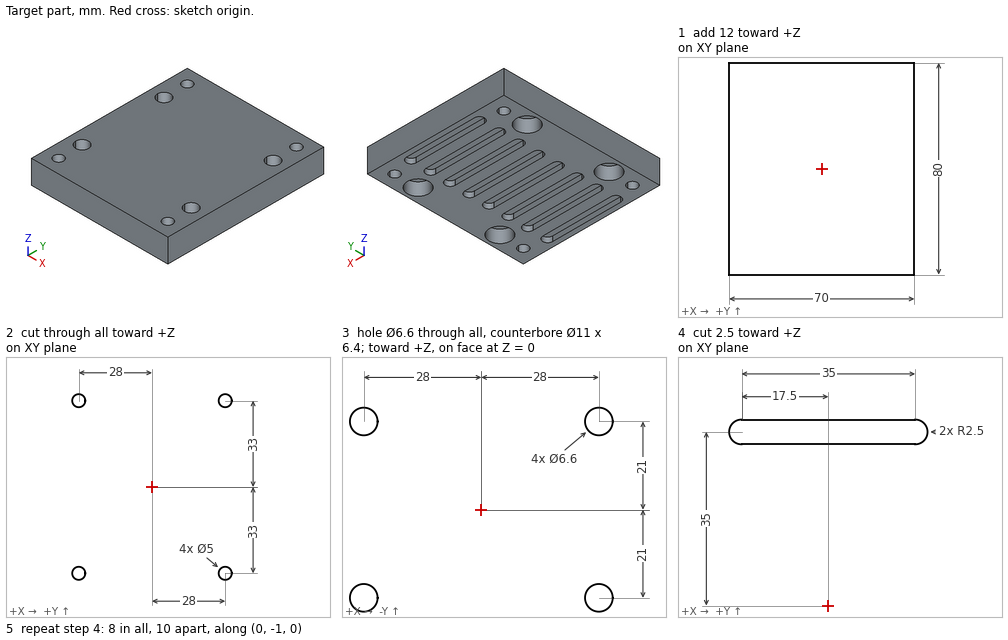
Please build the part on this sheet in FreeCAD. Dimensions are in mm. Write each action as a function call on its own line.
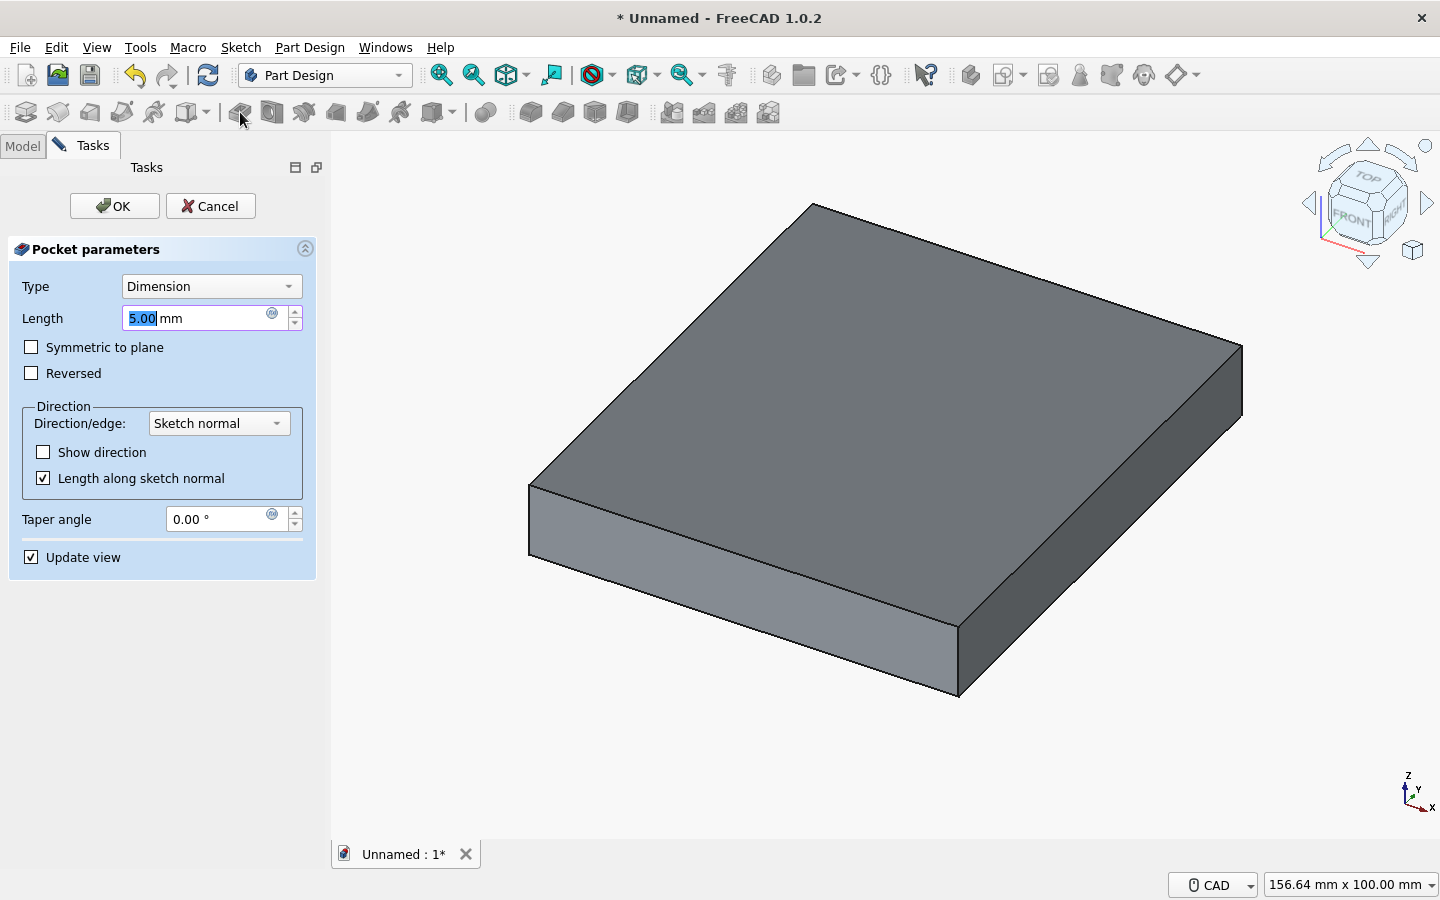
click(212, 286)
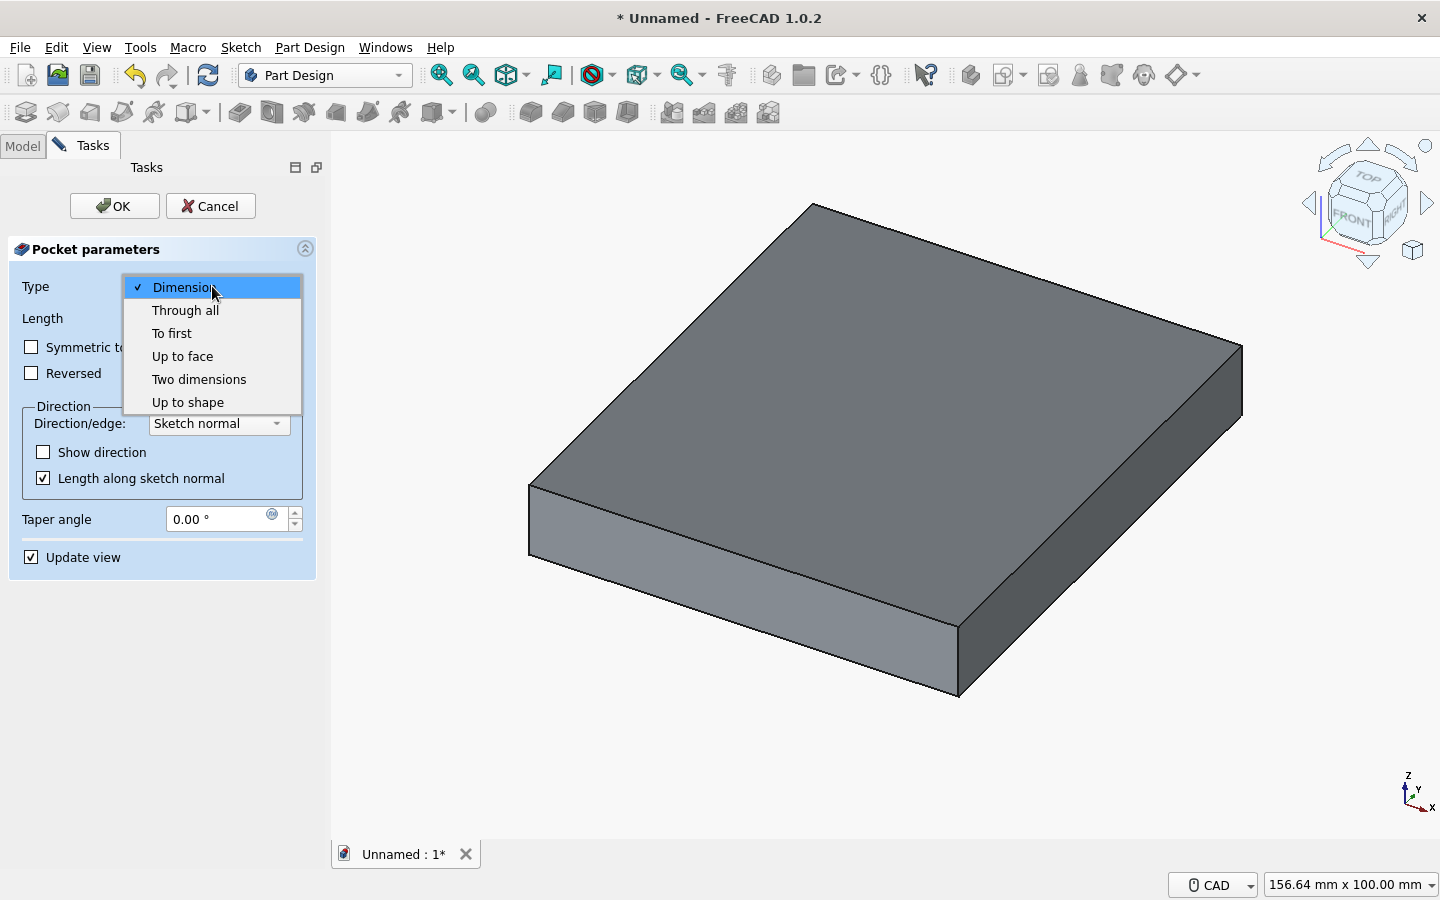
click(212, 310)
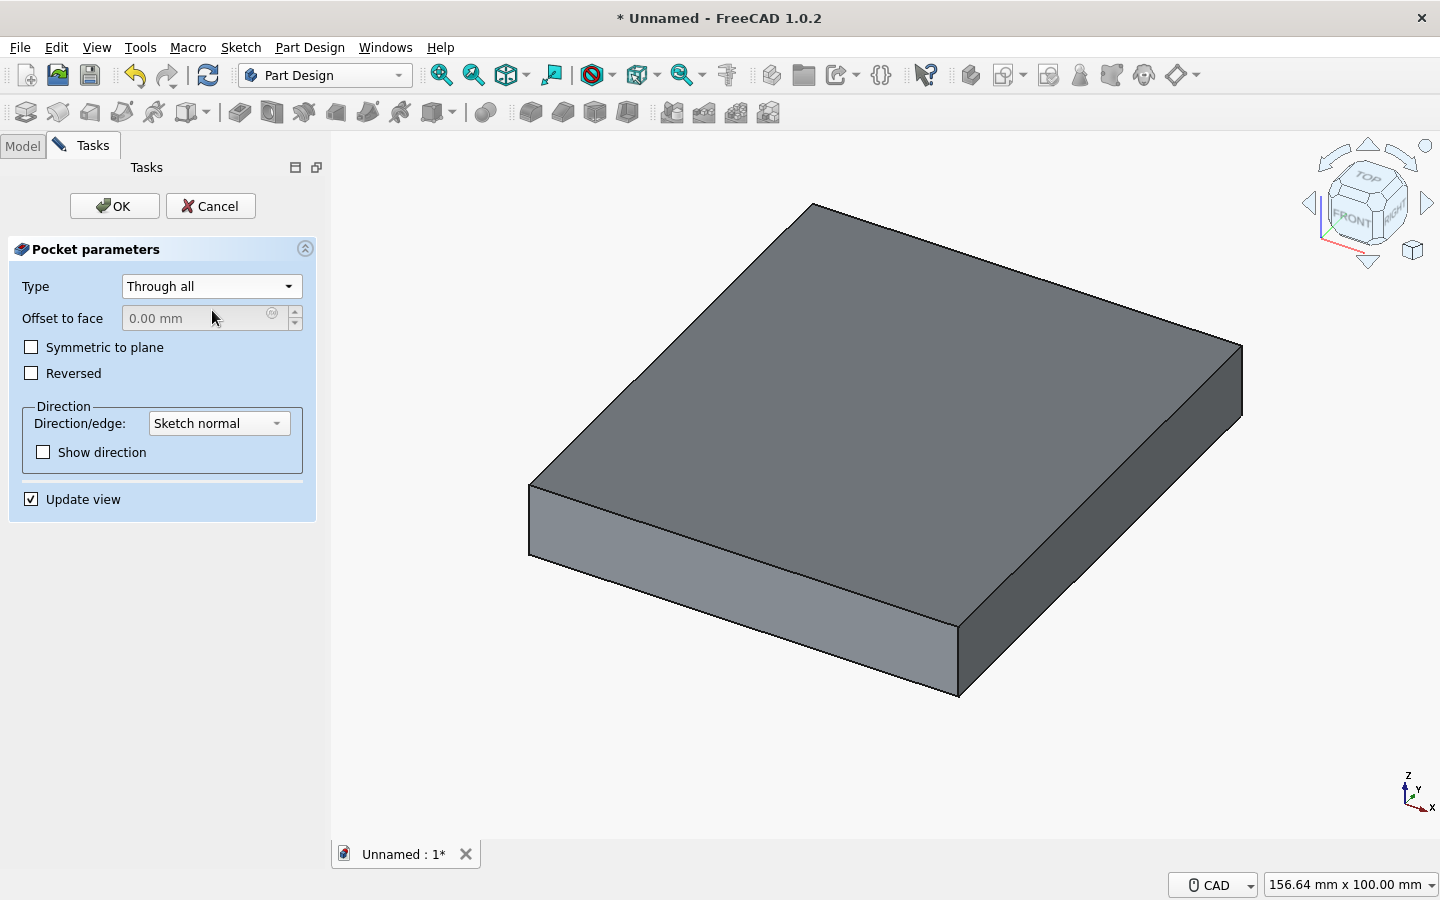
click(30, 373)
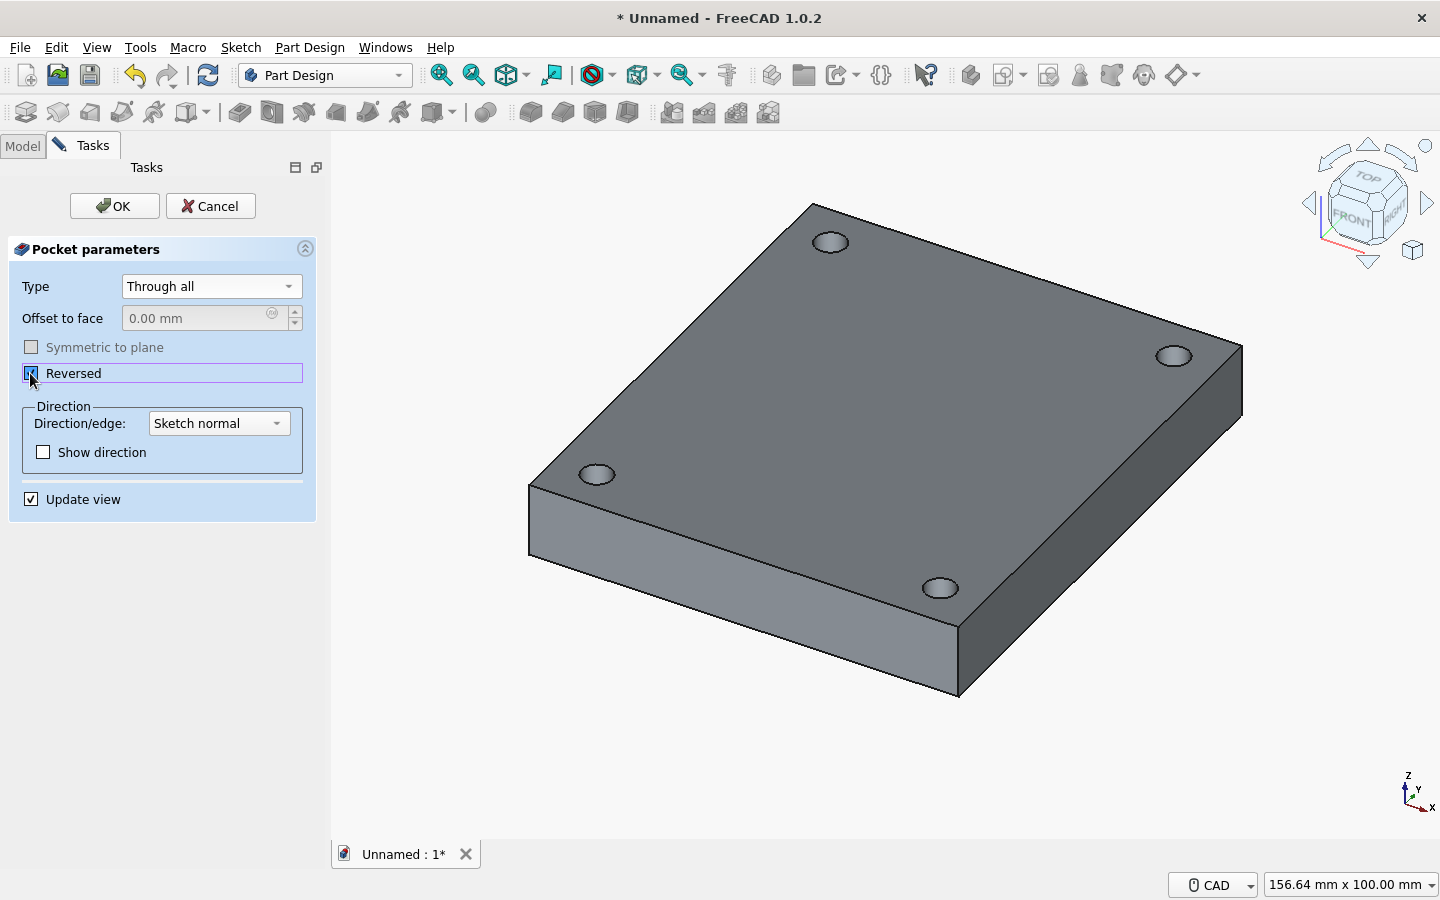
click(115, 206)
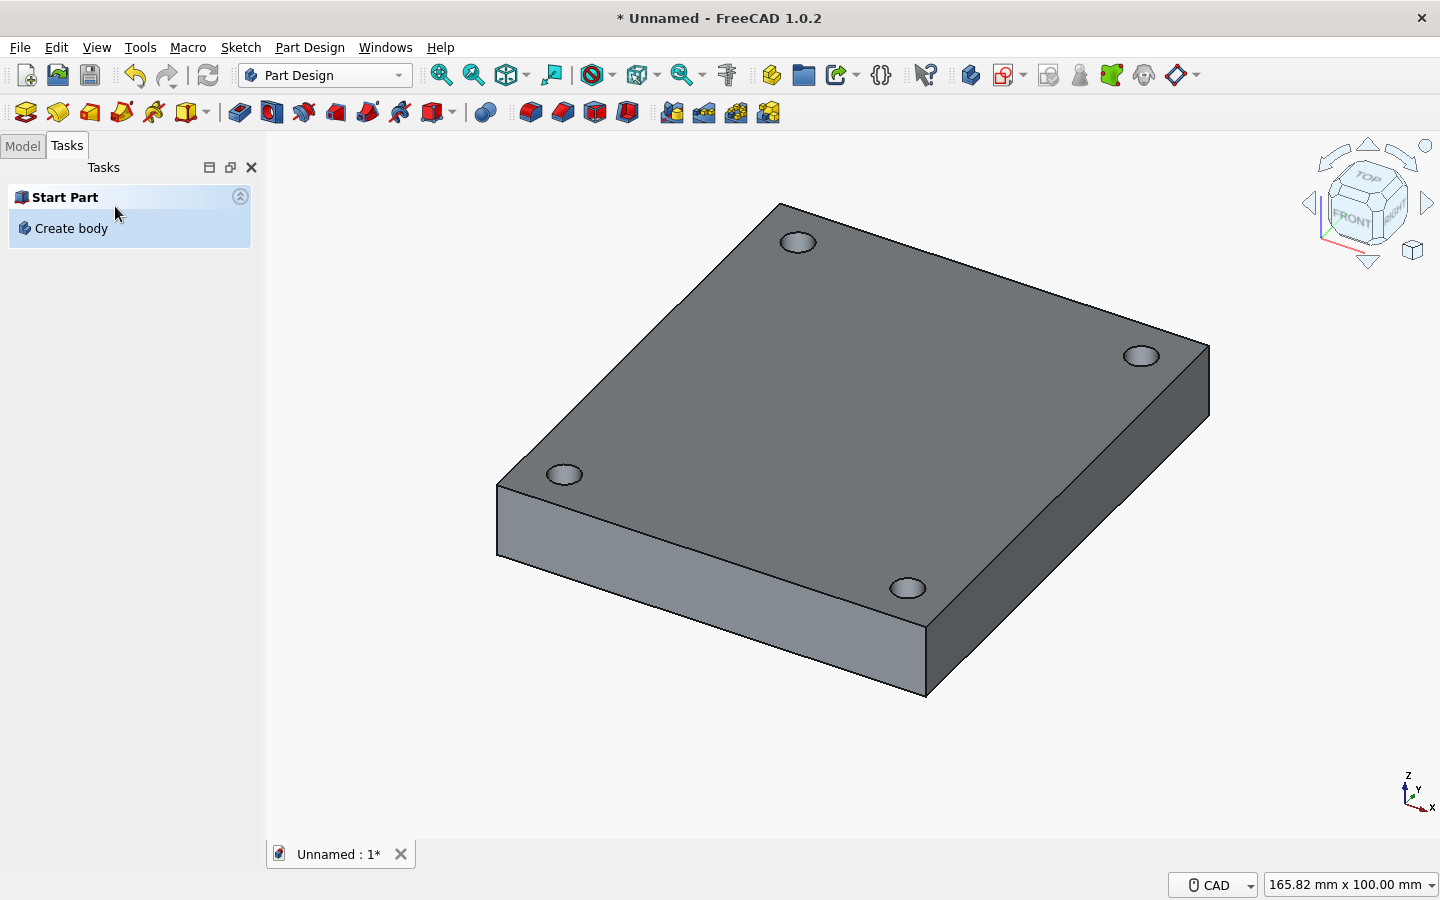
key(5)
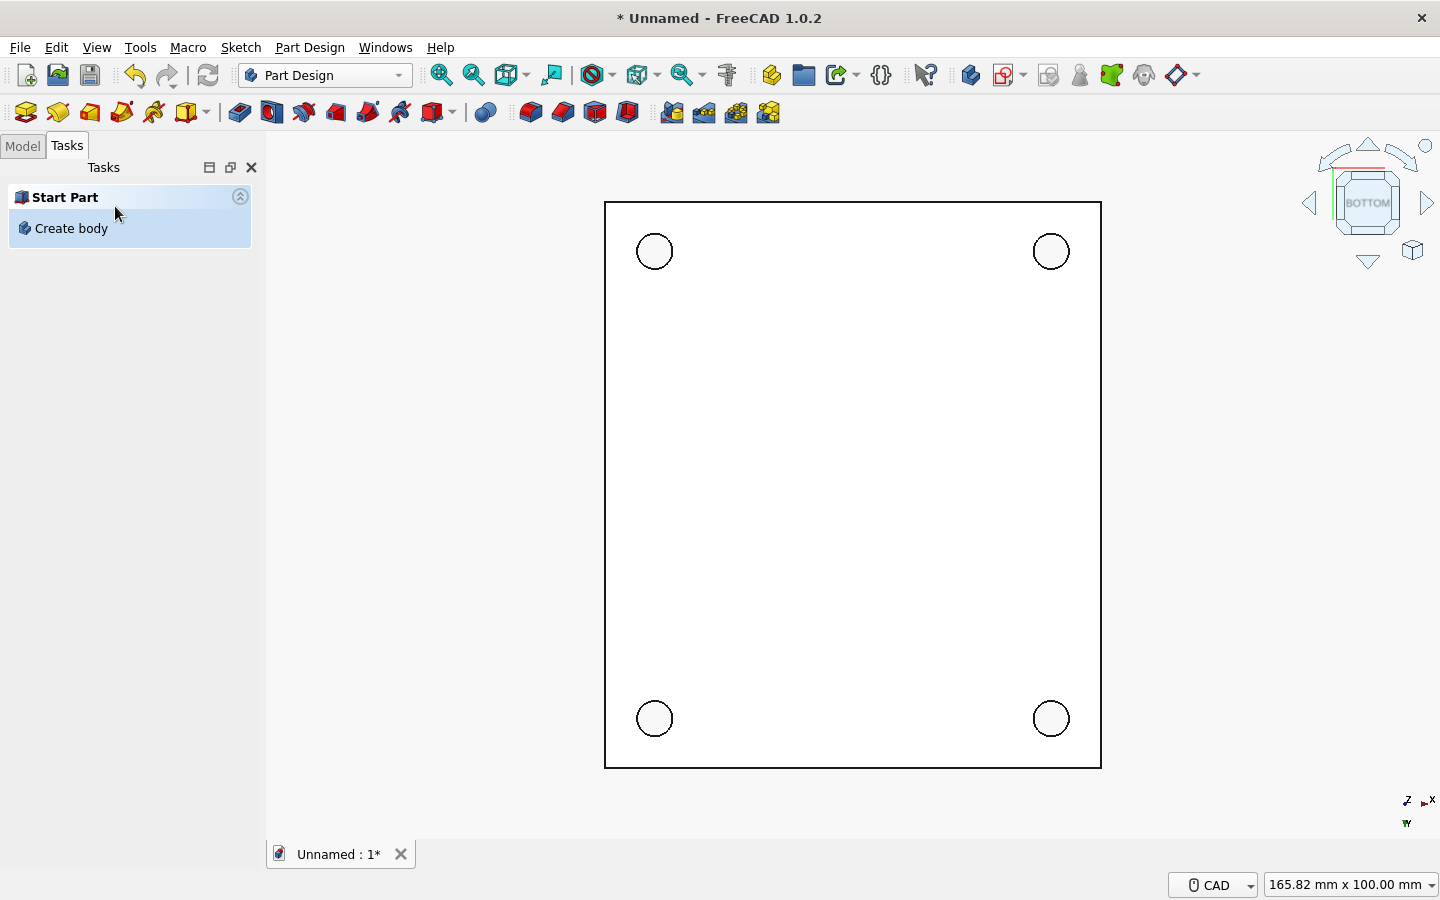
click(853, 484)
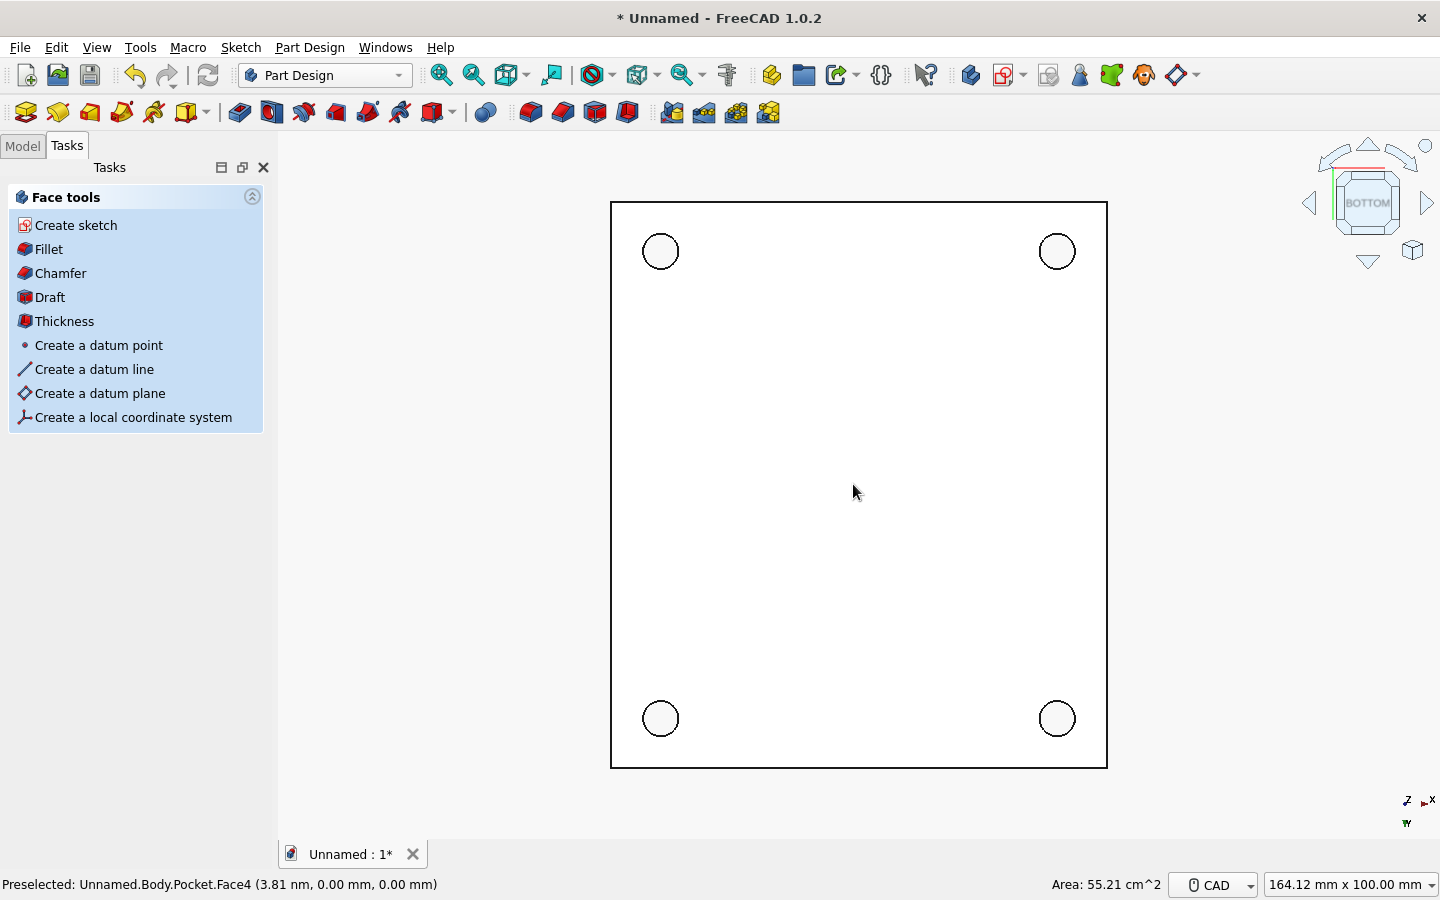
click(1004, 76)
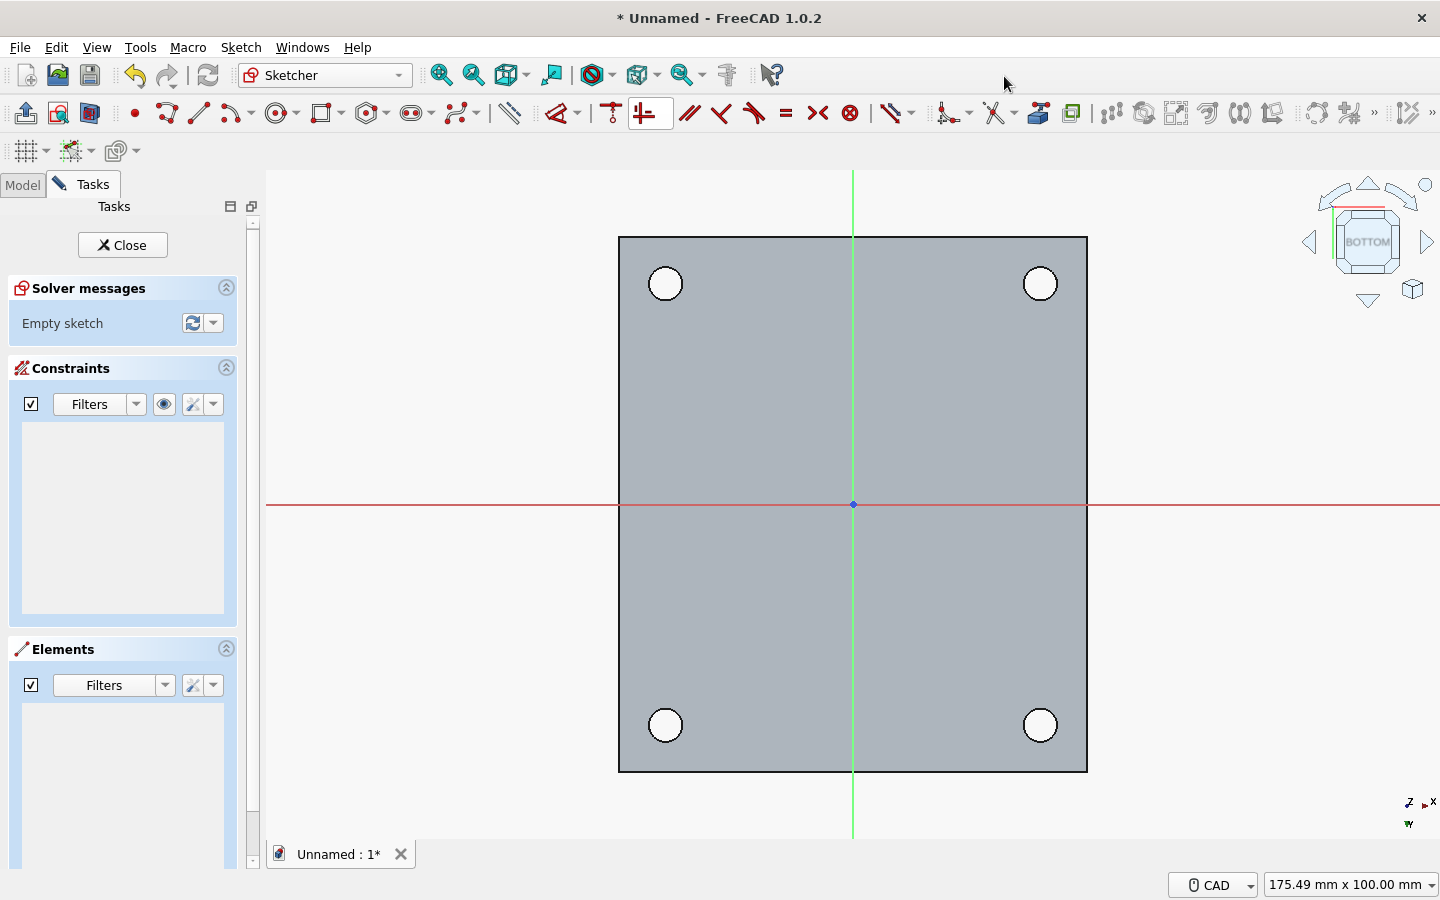
click(276, 114)